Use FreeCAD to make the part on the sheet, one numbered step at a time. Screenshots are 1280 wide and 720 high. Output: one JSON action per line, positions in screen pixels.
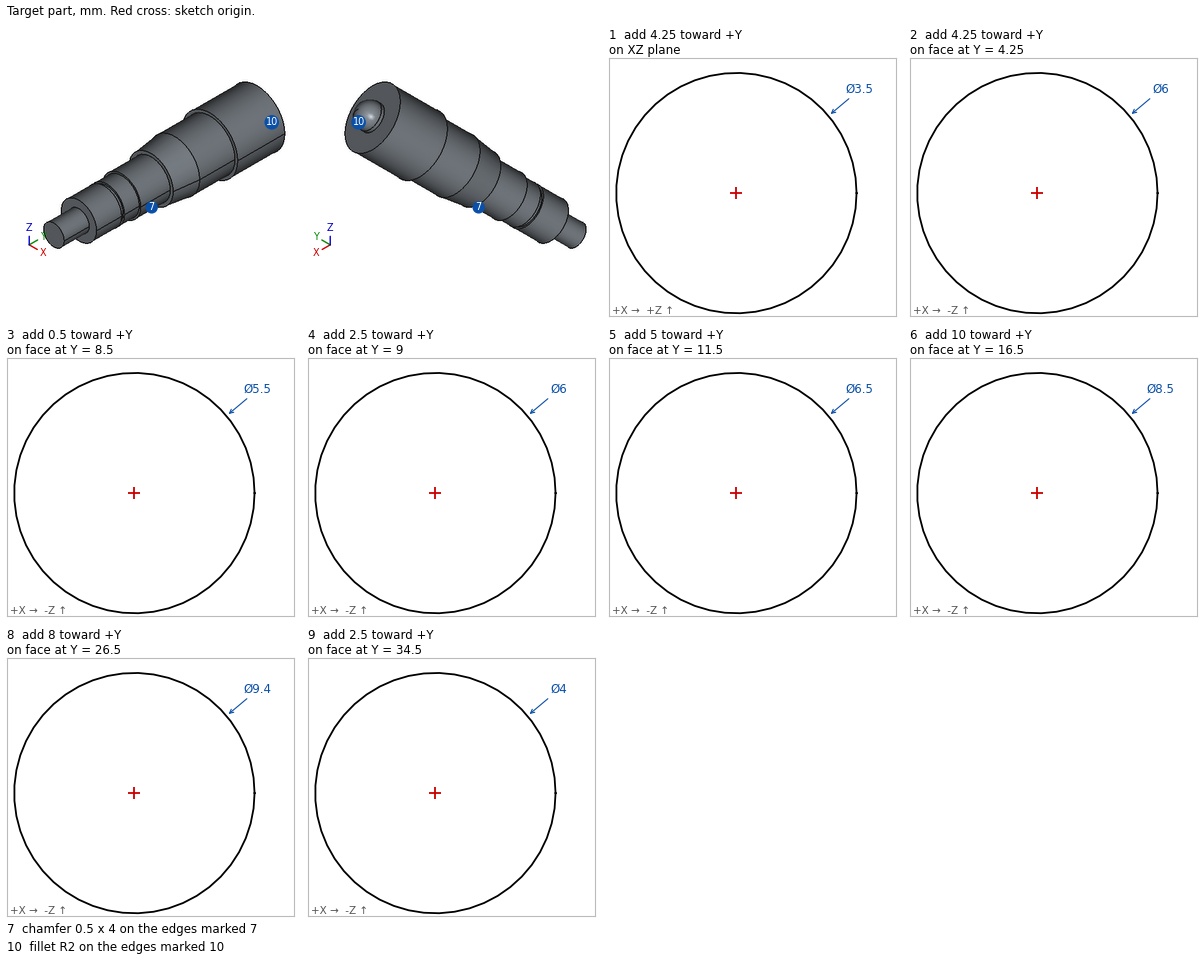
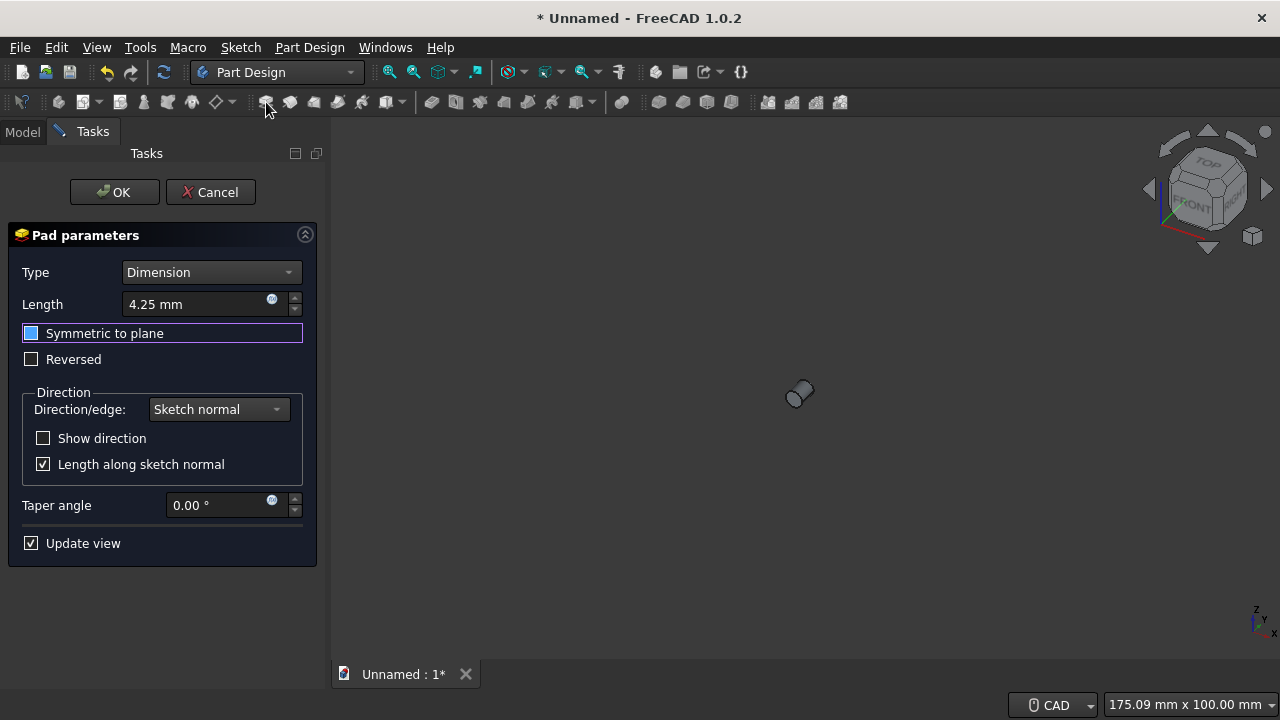
{"action": "left_click", "coordinate": [30, 359]}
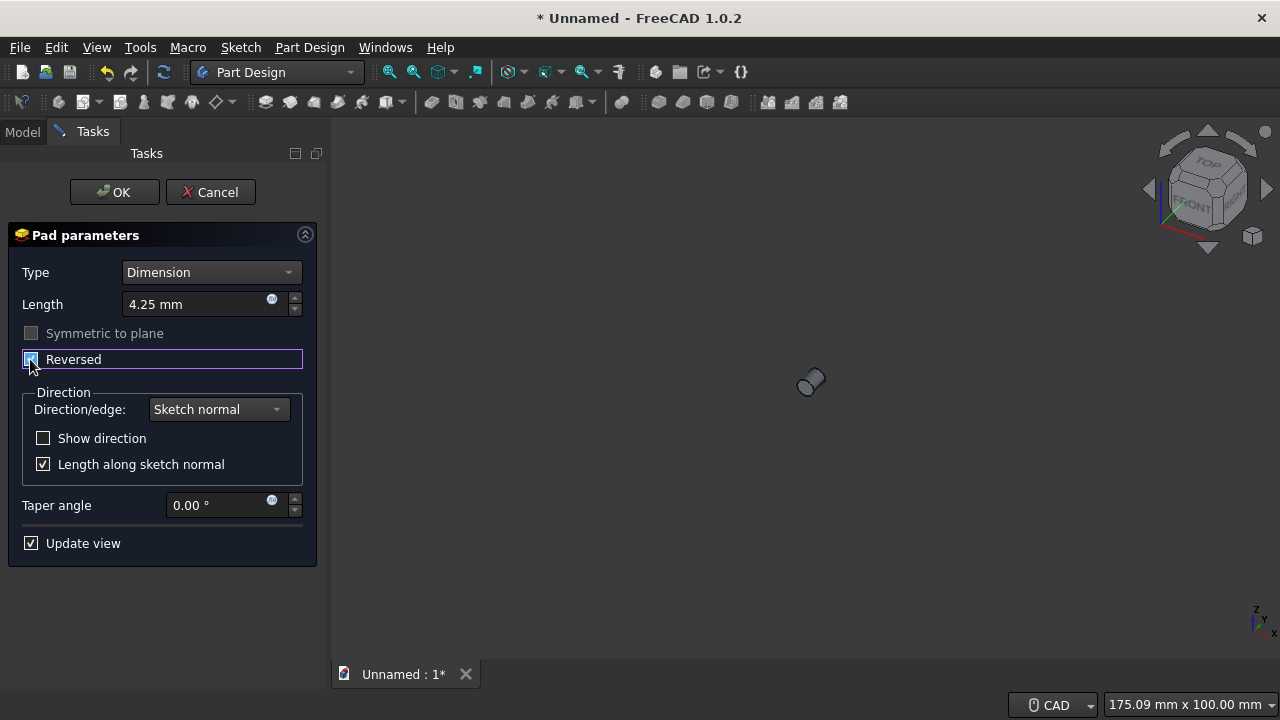
{"action": "left_click", "coordinate": [115, 192]}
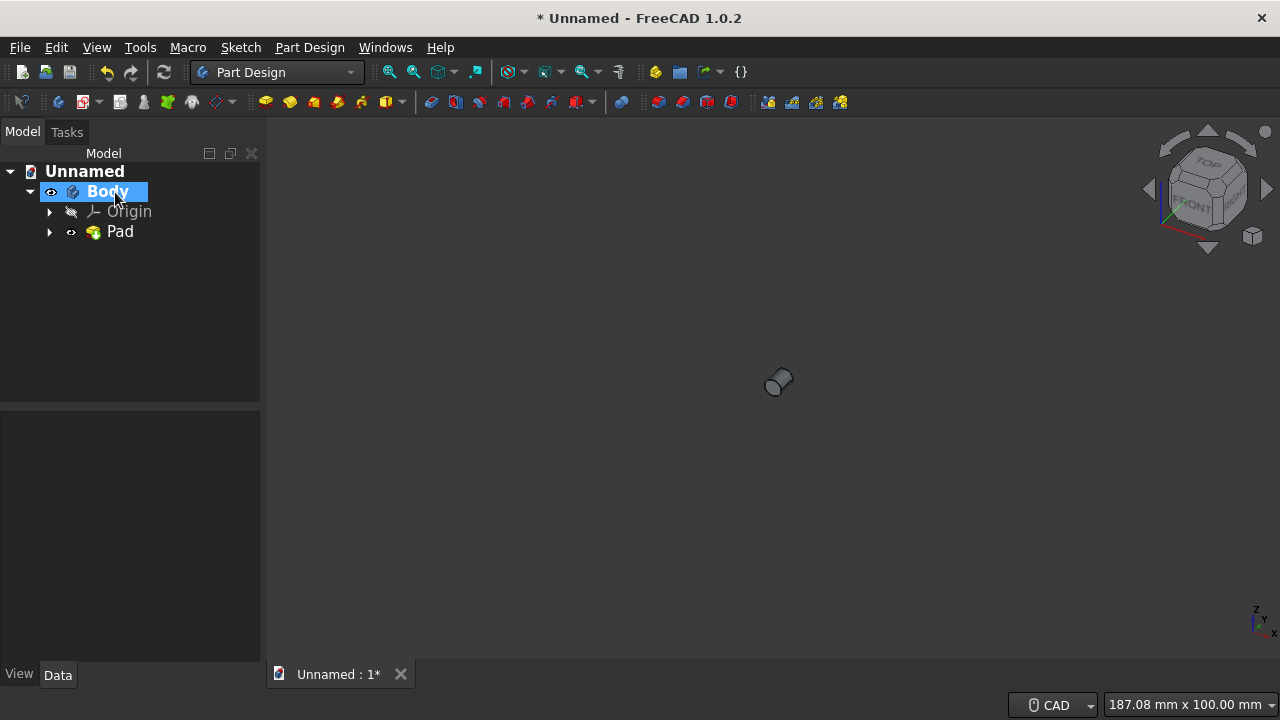
{"action": "left_click", "coordinate": [390, 72]}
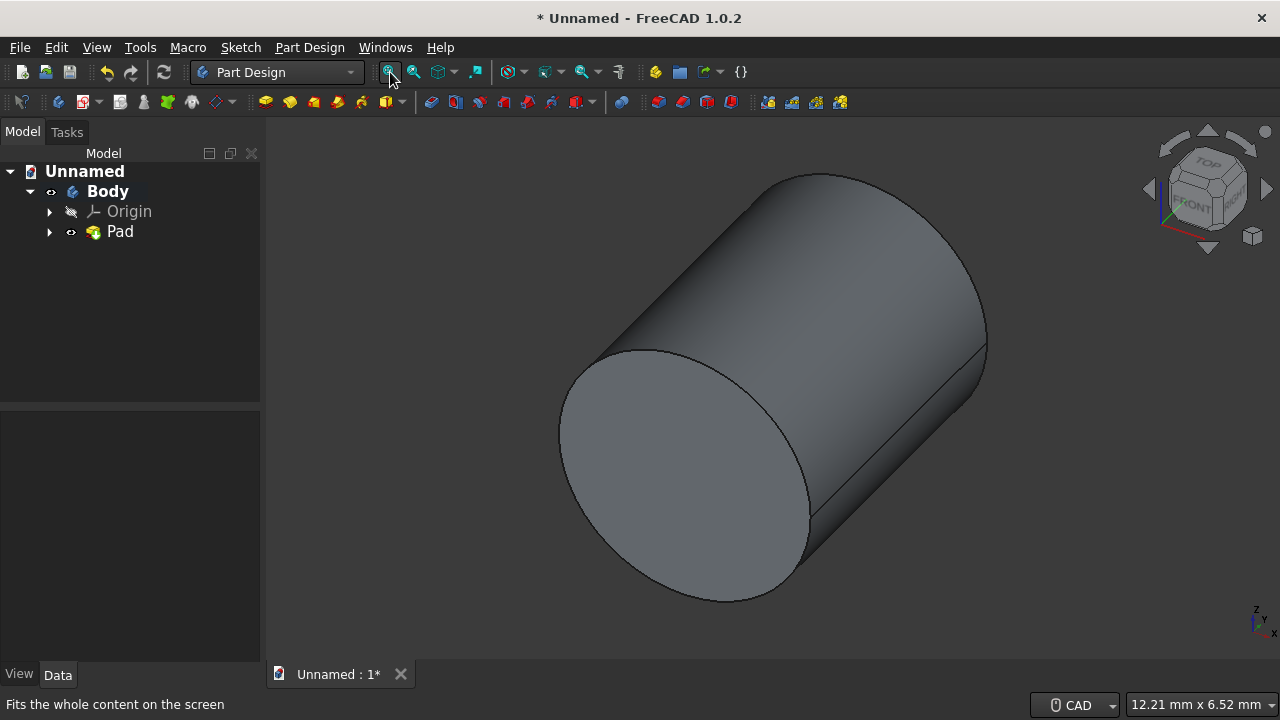
{"action": "key", "text": "4"}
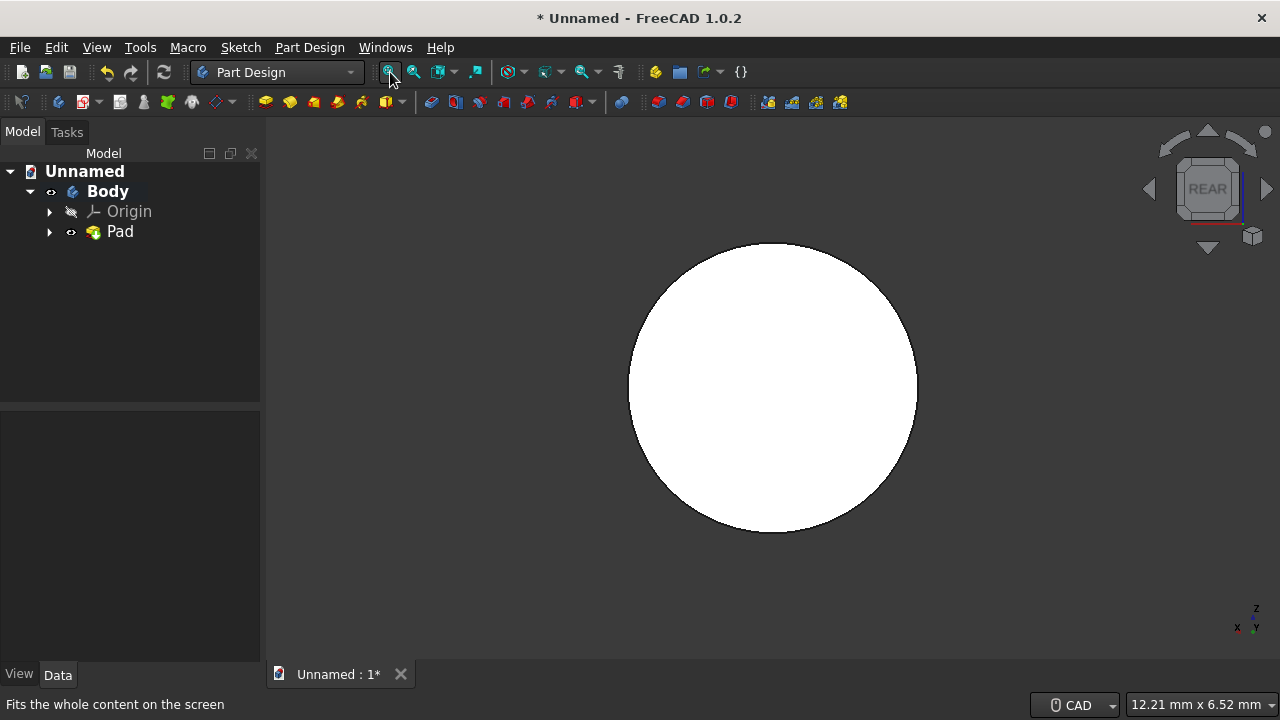
{"action": "left_click", "coordinate": [773, 387]}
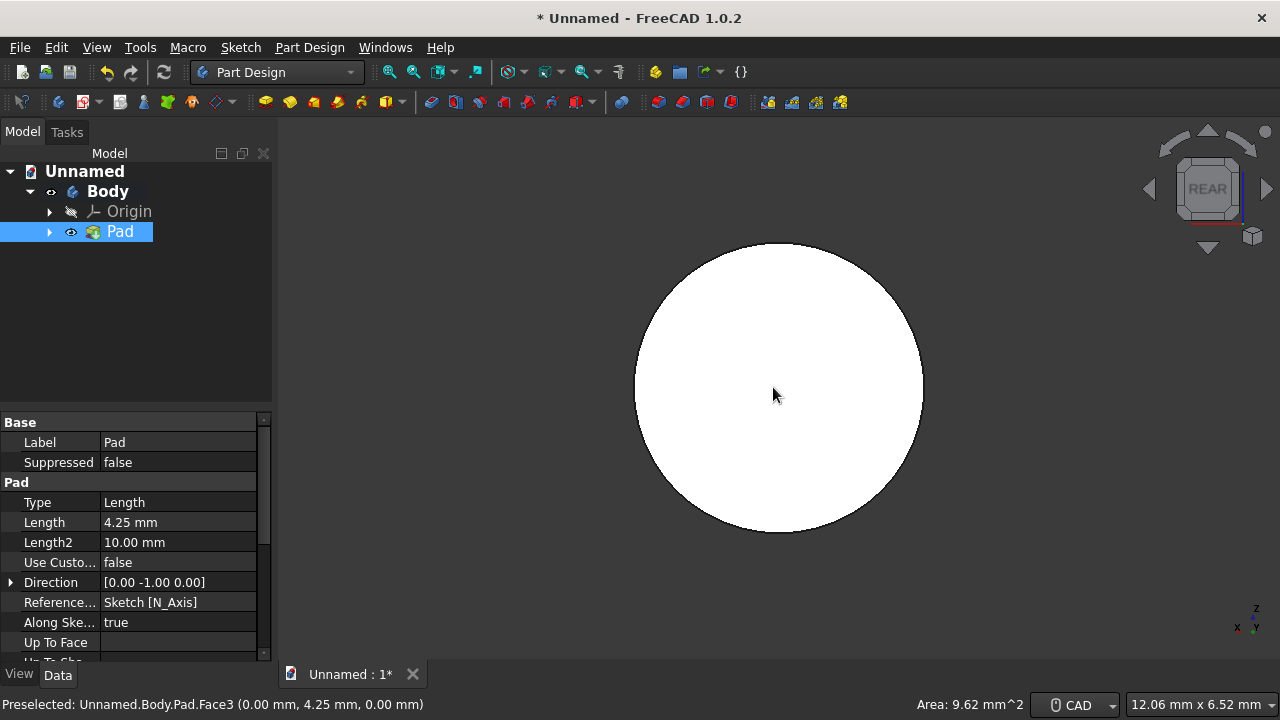
{"action": "left_click", "coordinate": [84, 102]}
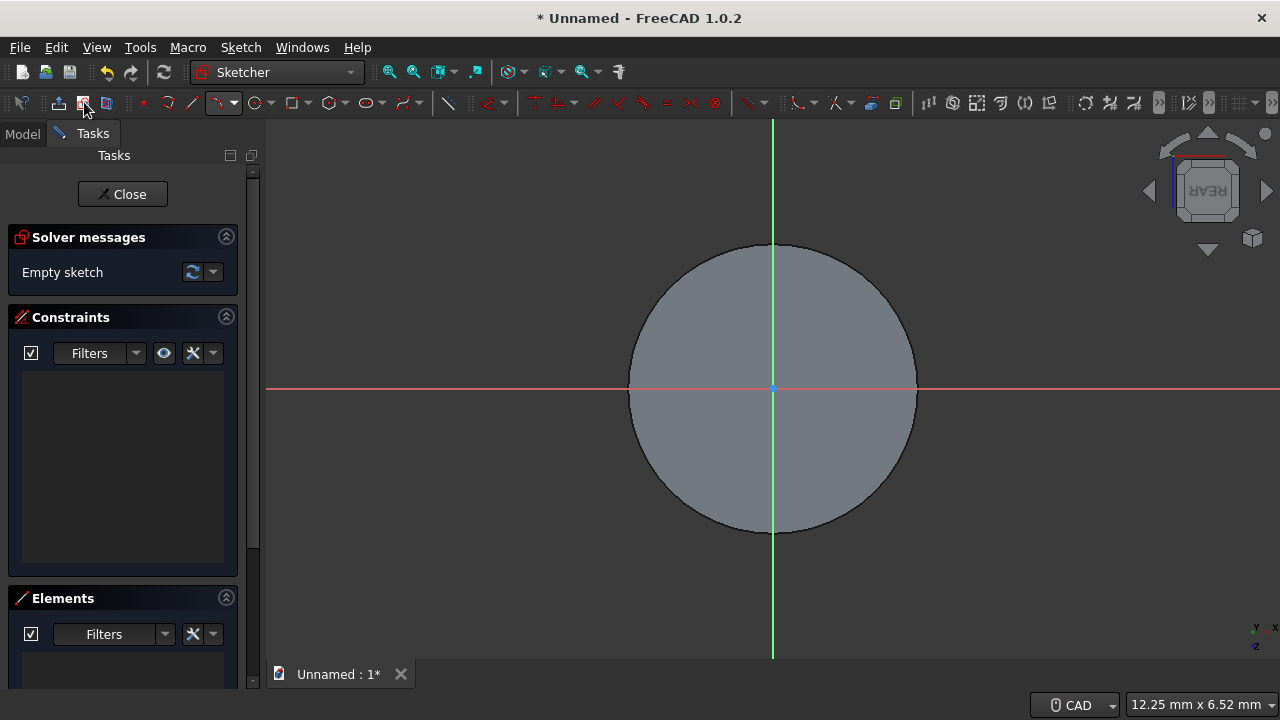
{"action": "scroll", "coordinate": [565, 389], "scroll_direction": "down", "scroll_amount": 2}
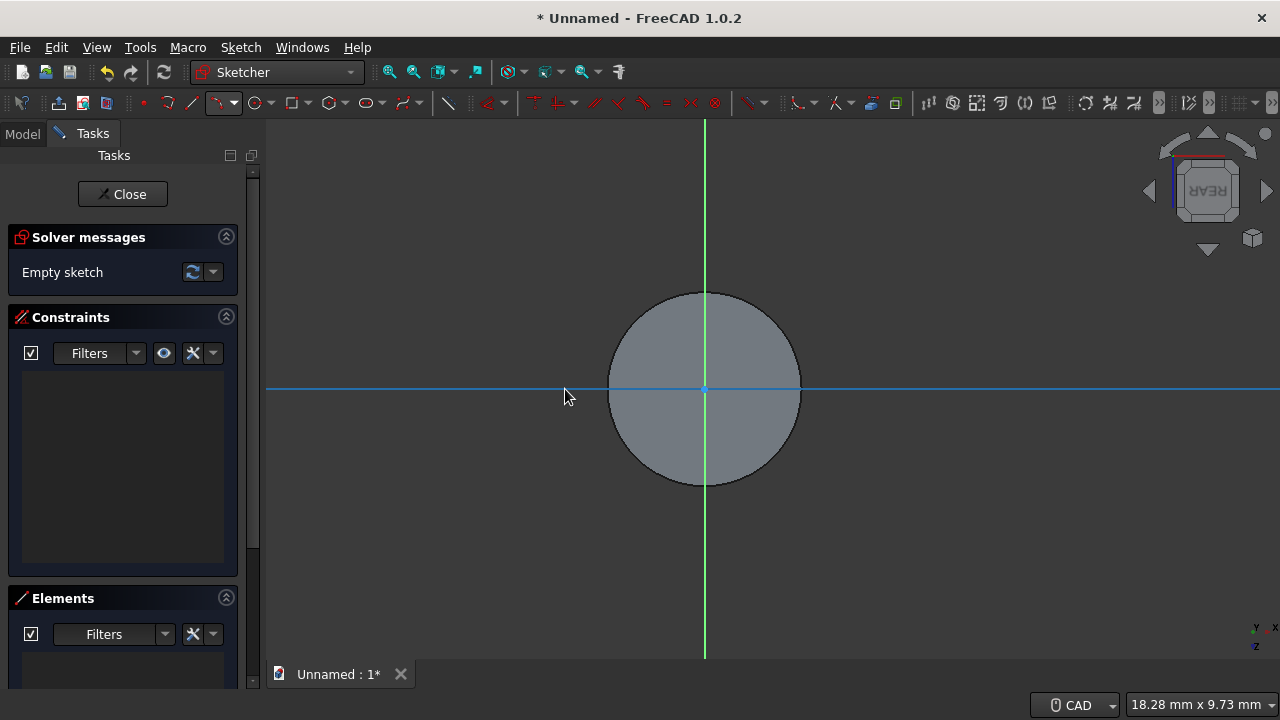
{"action": "left_click", "coordinate": [256, 104]}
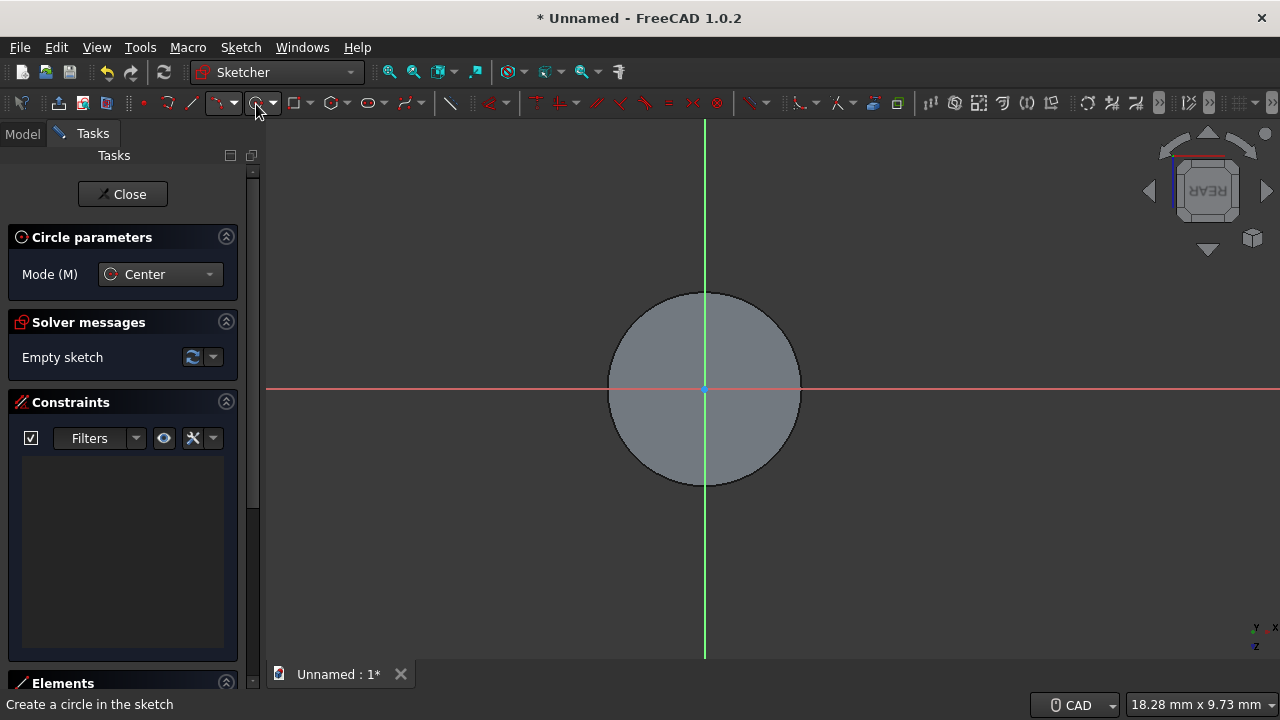
{"action": "left_click", "coordinate": [705, 389]}
{"action": "mouse_move", "coordinate": [822, 271]}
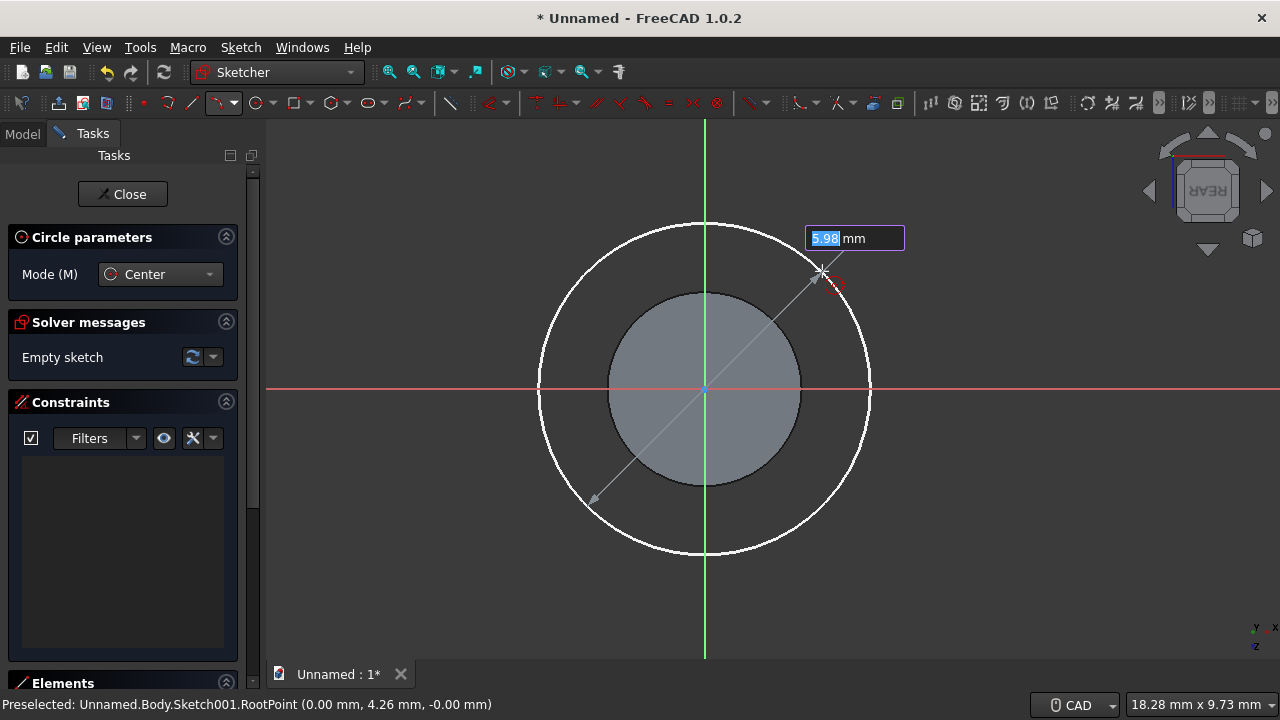
{"action": "type", "text": "6"}
{"action": "key", "text": "Return"}
{"action": "key", "text": "Escape"}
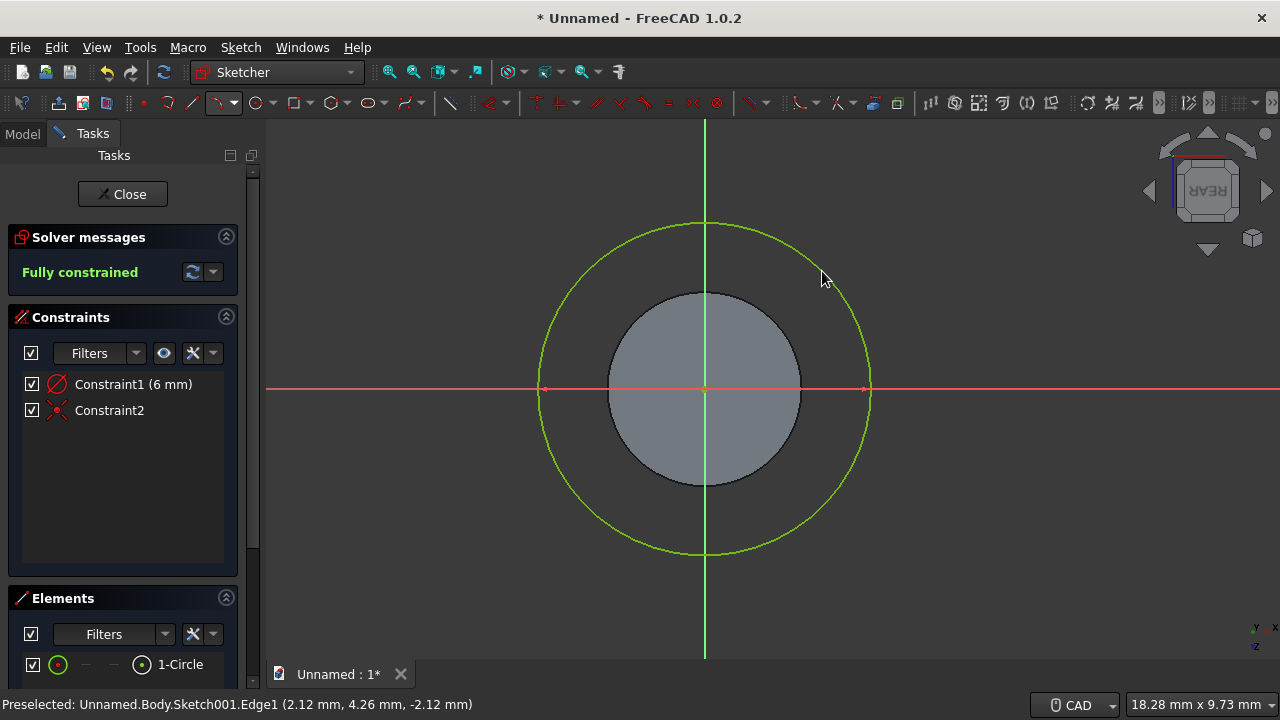
{"action": "left_click", "coordinate": [123, 194]}